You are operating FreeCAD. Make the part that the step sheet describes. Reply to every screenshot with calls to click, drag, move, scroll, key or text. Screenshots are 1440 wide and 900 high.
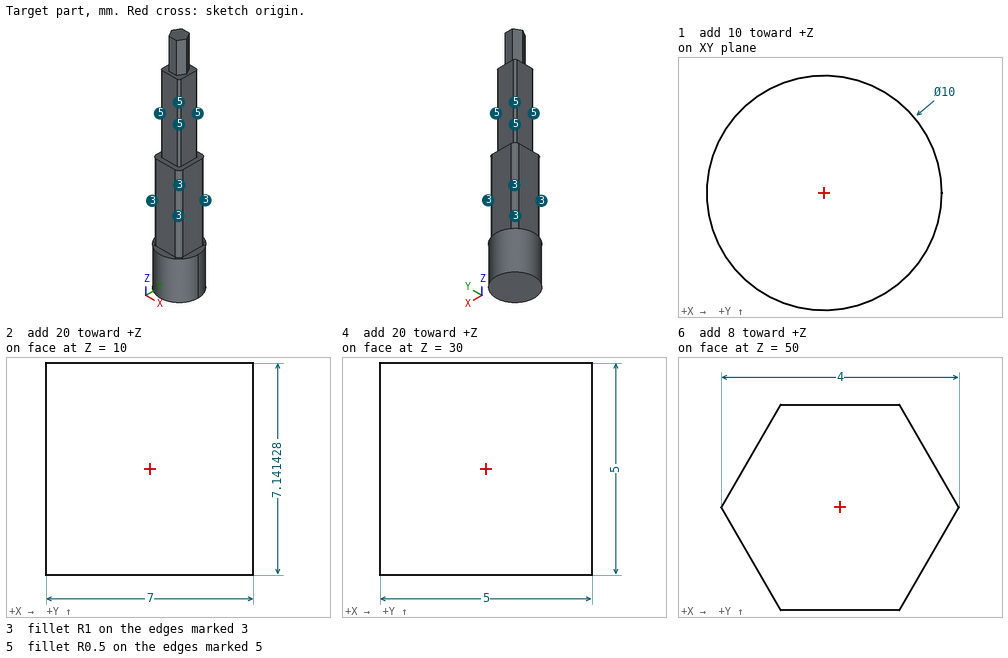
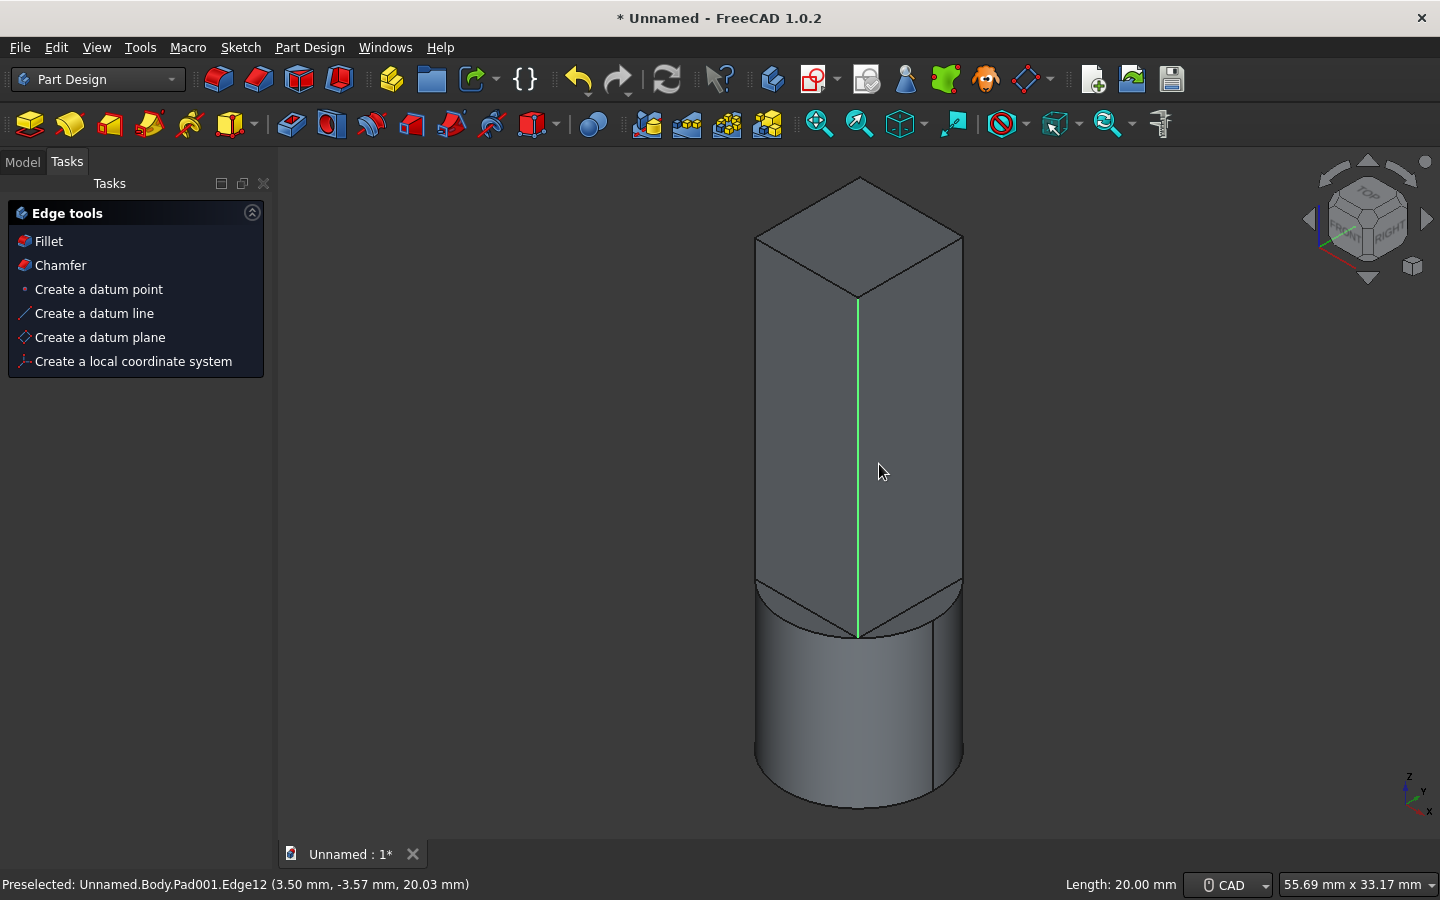
key(2)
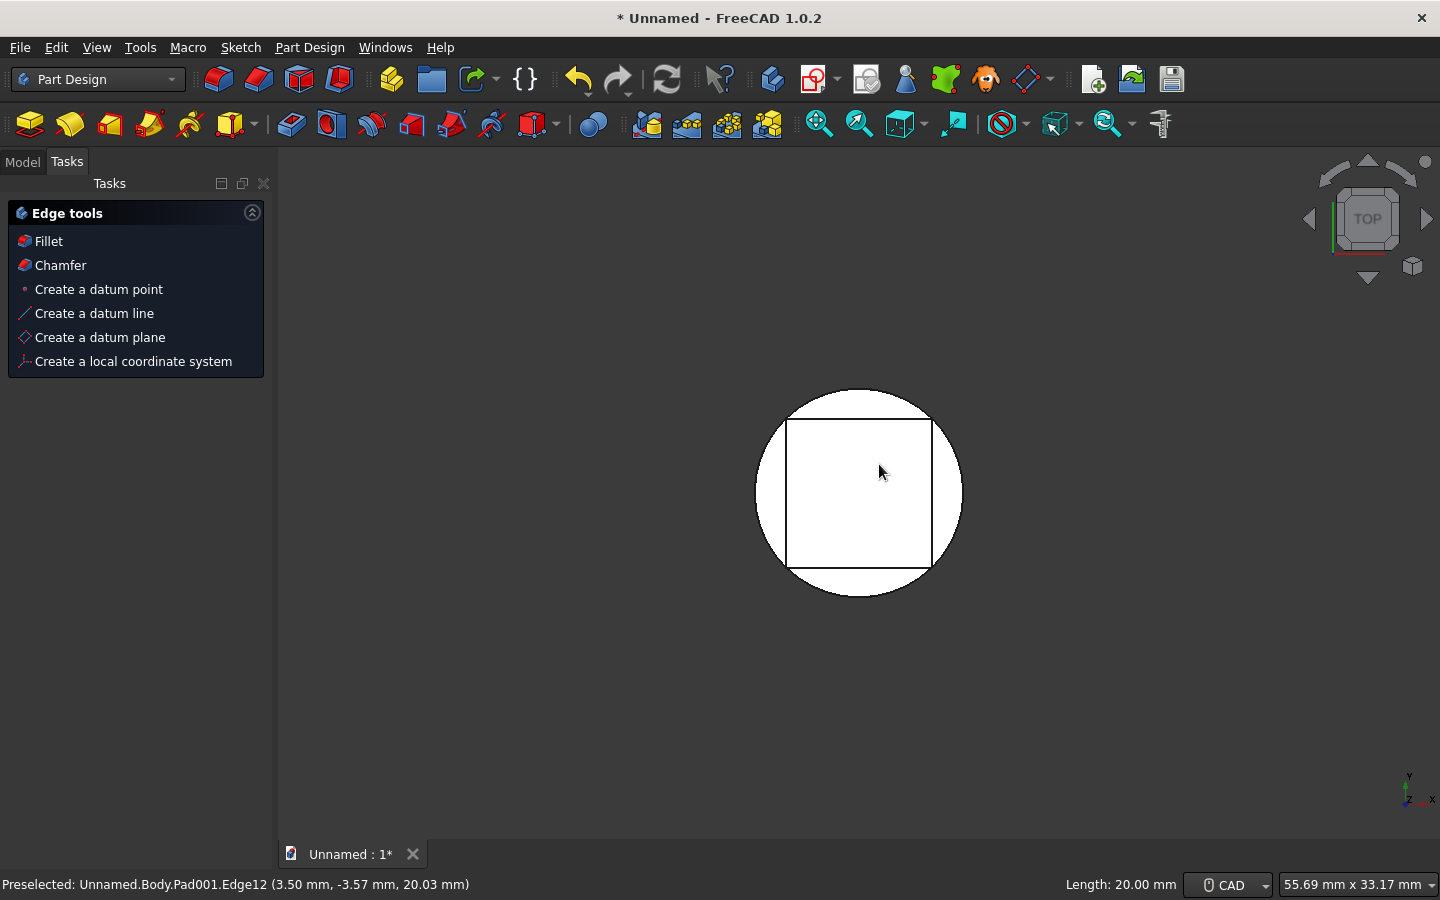
click(820, 124)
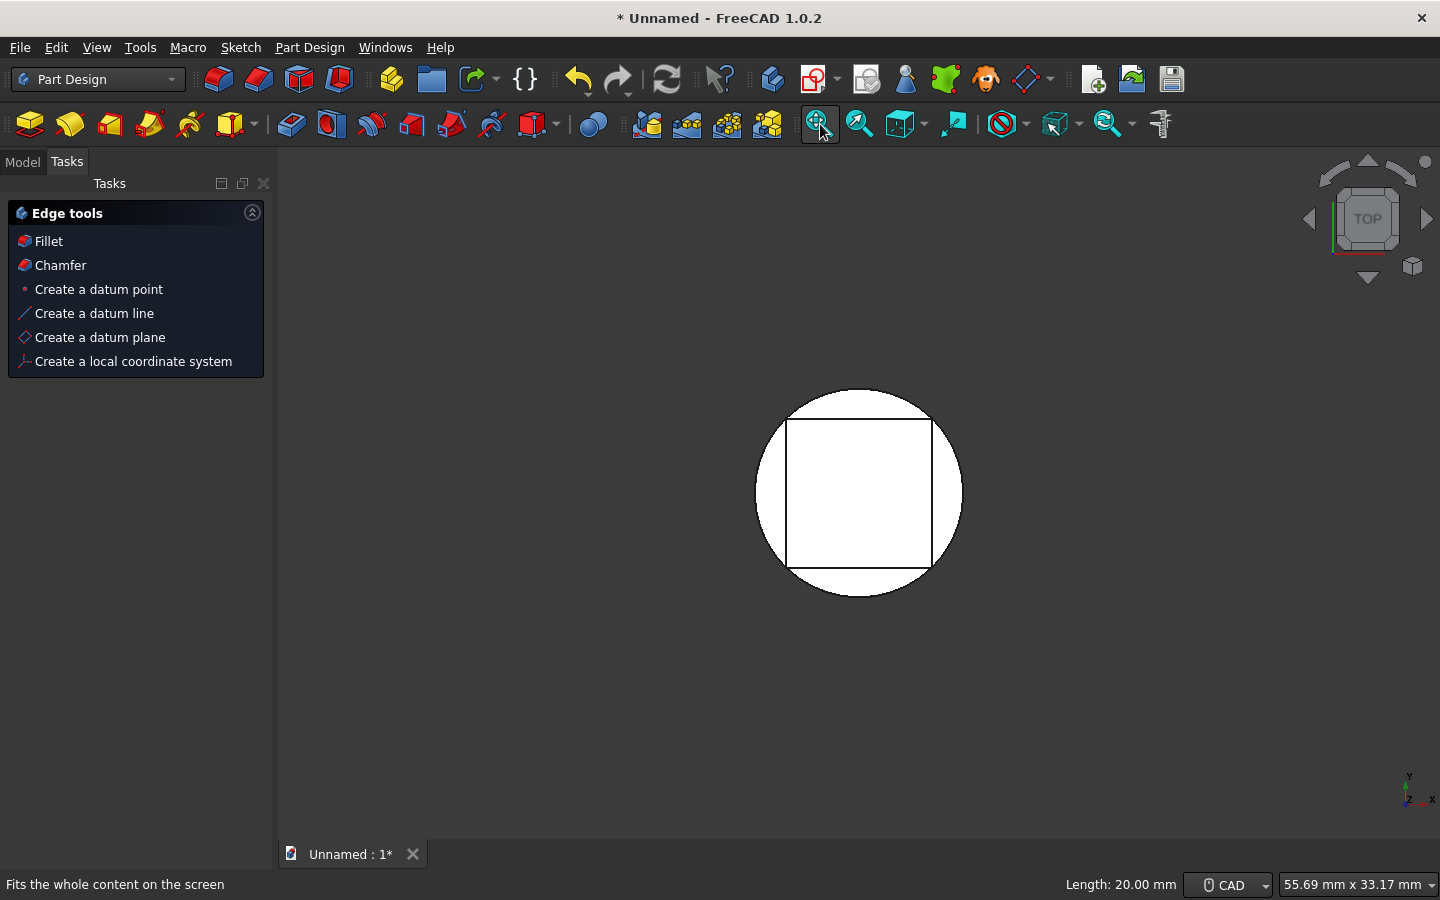
key(1)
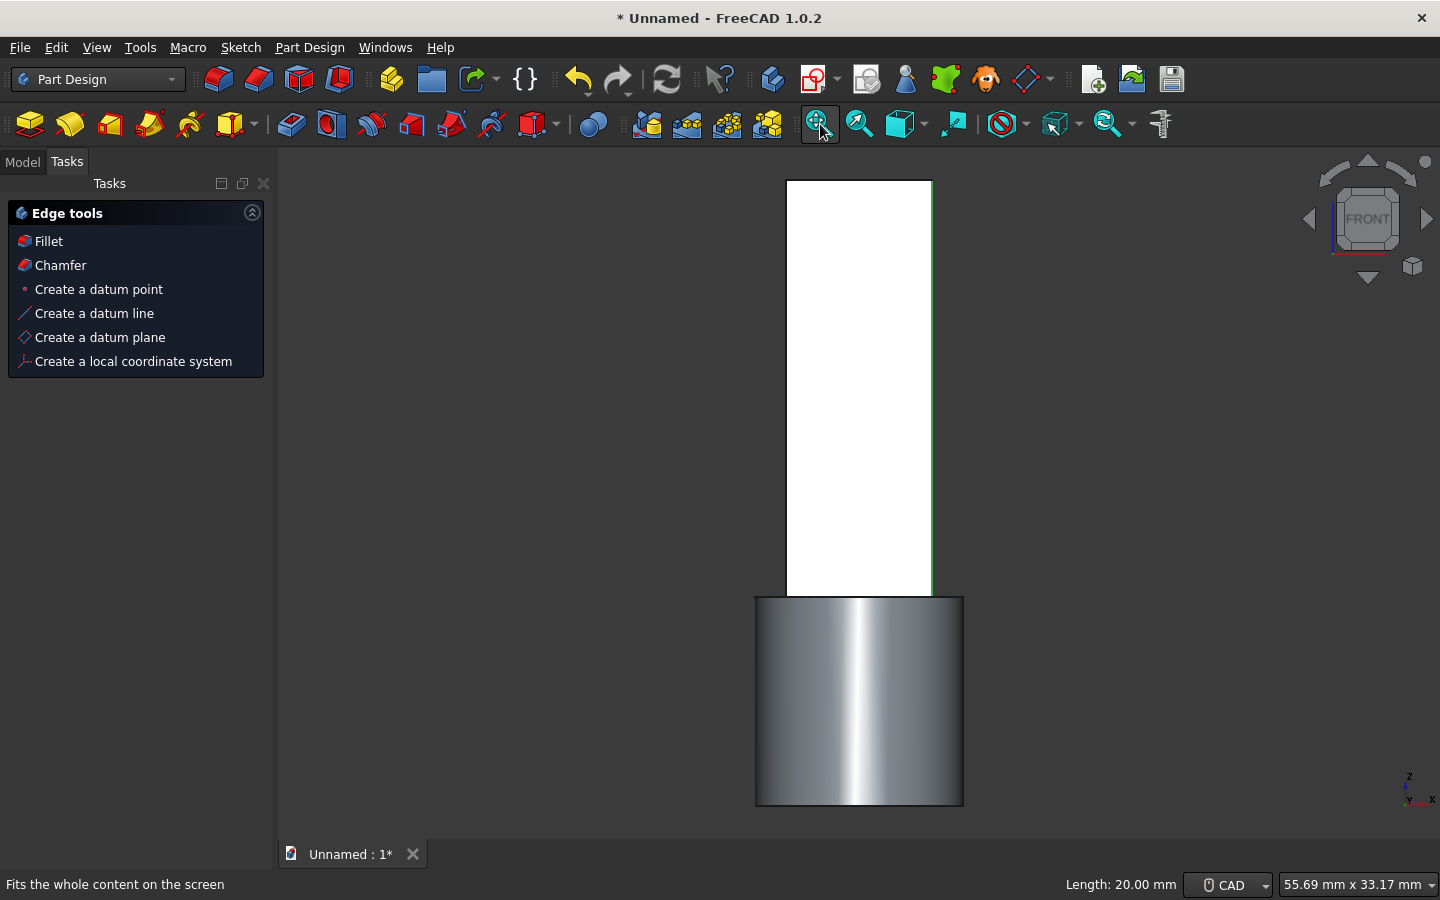
click(786, 388, ctrl)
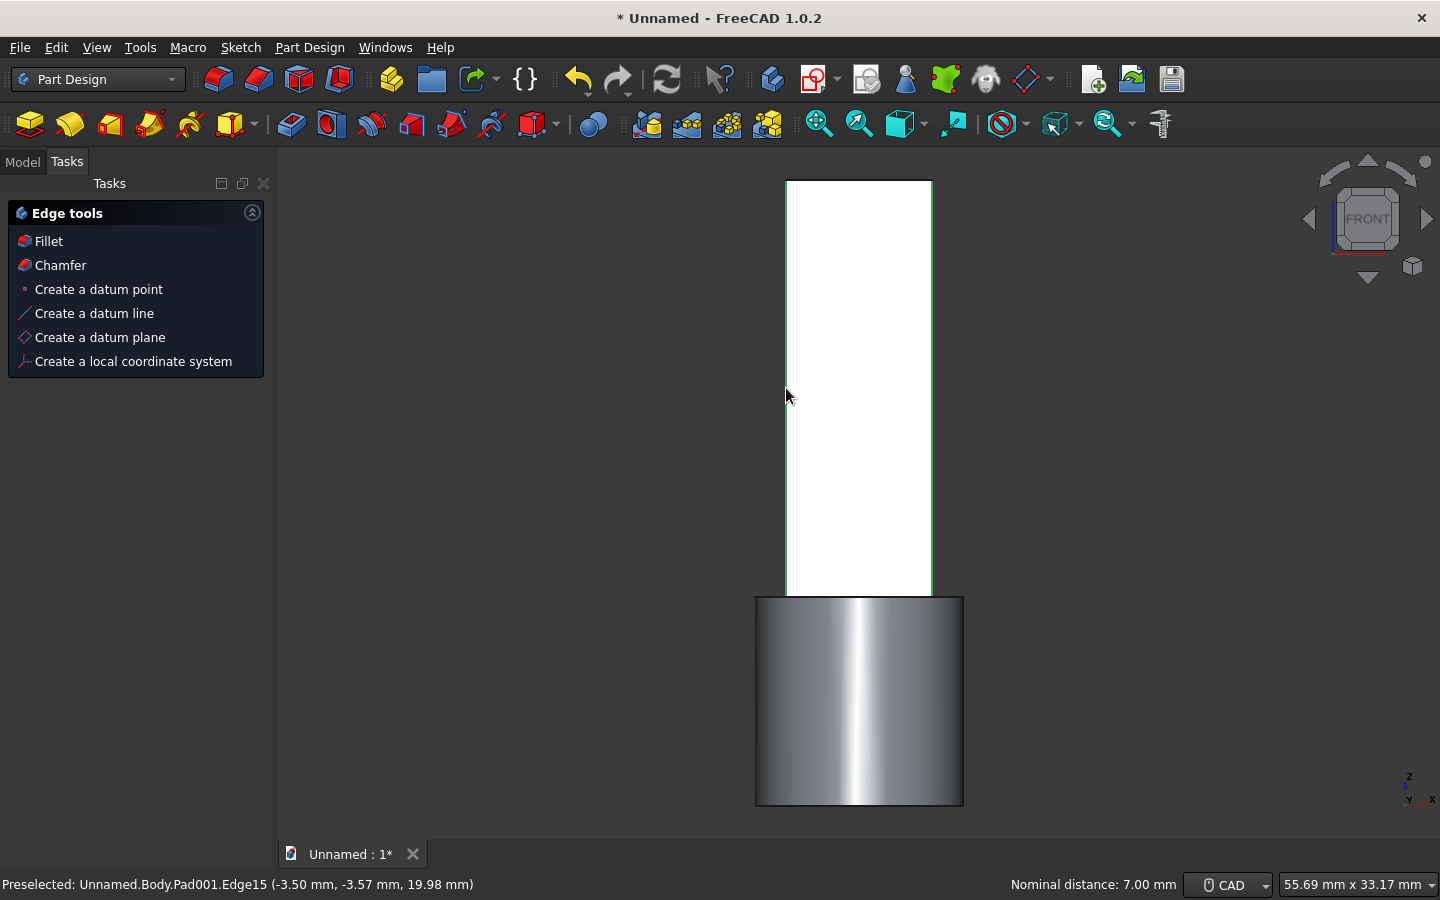
key(3)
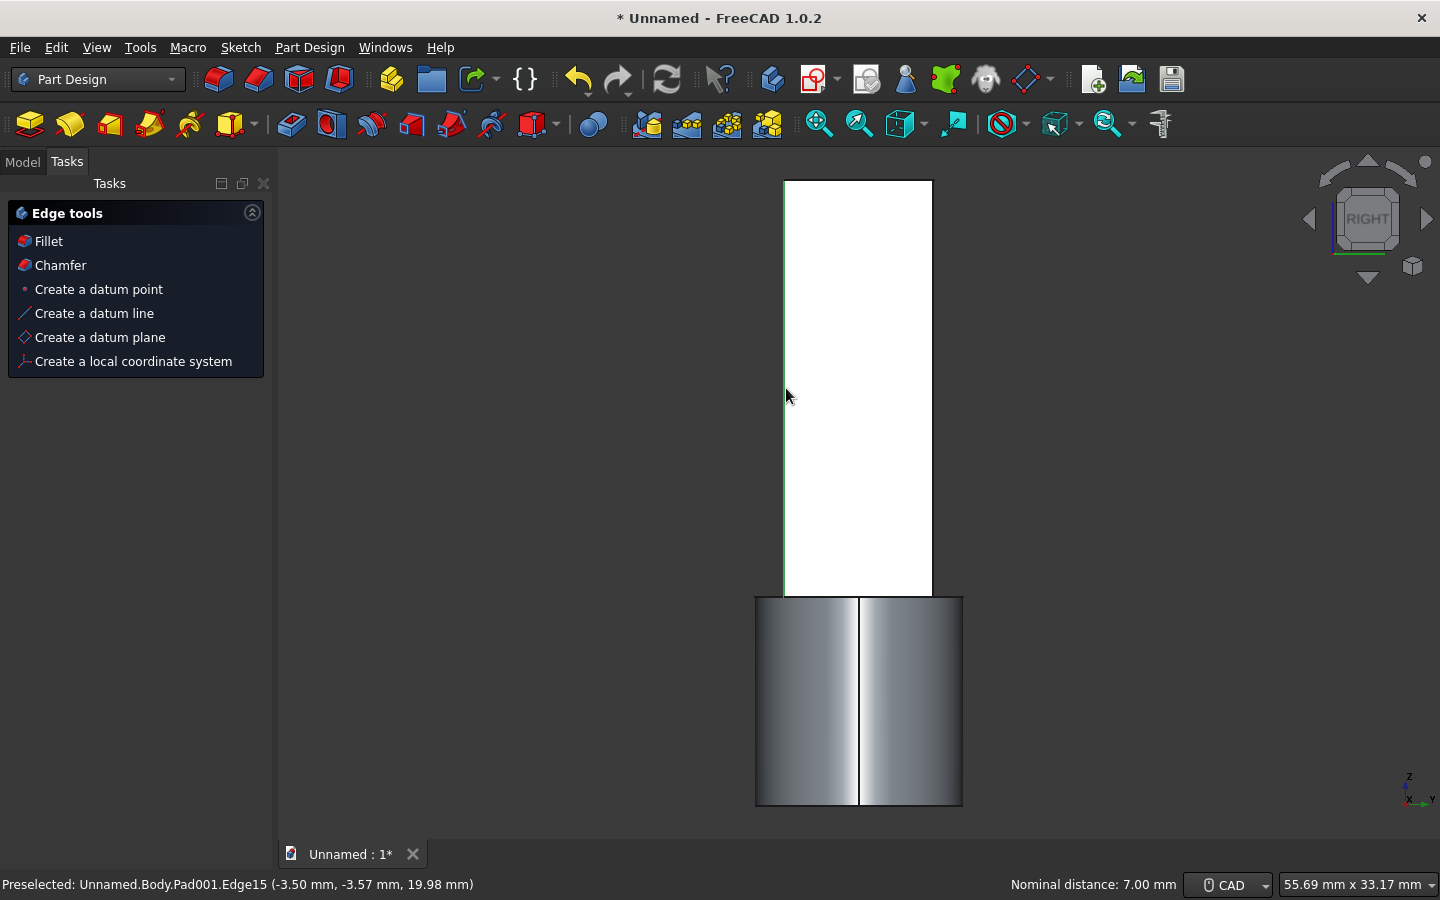
click(934, 388, ctrl)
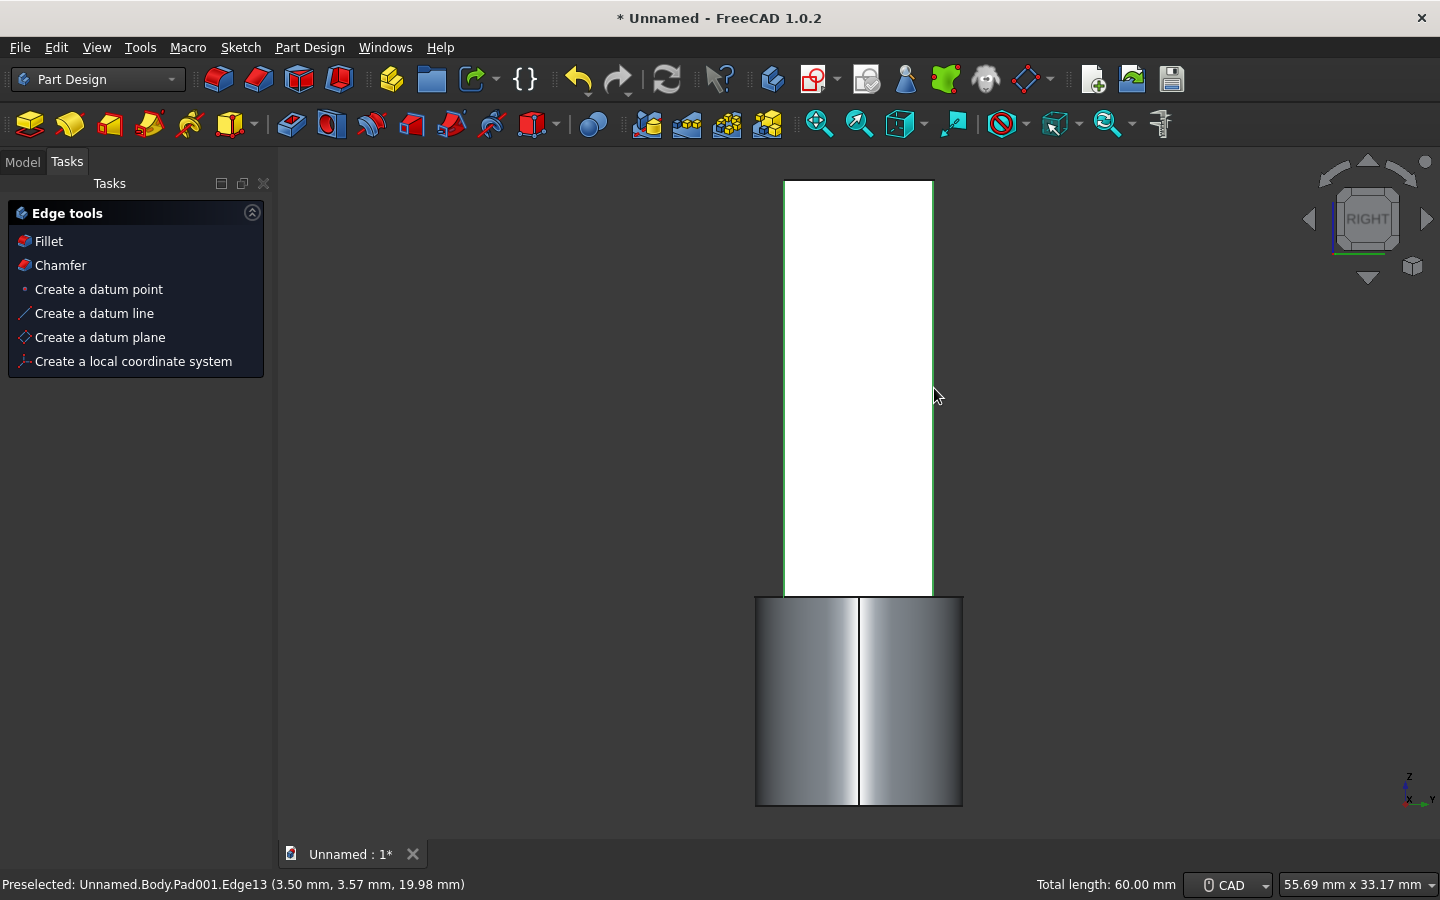
key(5)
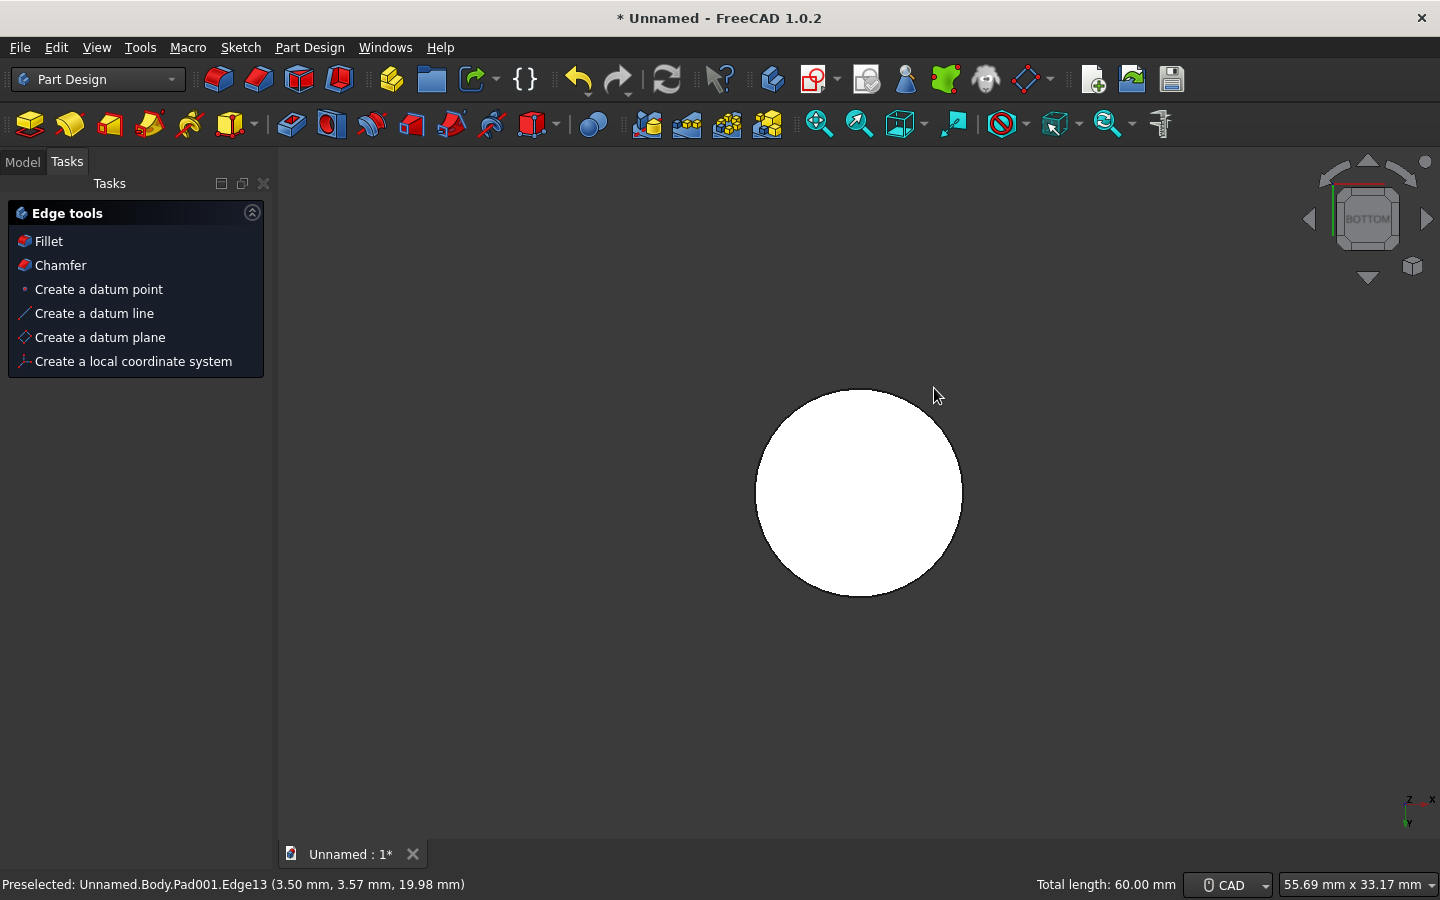
key(v)
key(f)